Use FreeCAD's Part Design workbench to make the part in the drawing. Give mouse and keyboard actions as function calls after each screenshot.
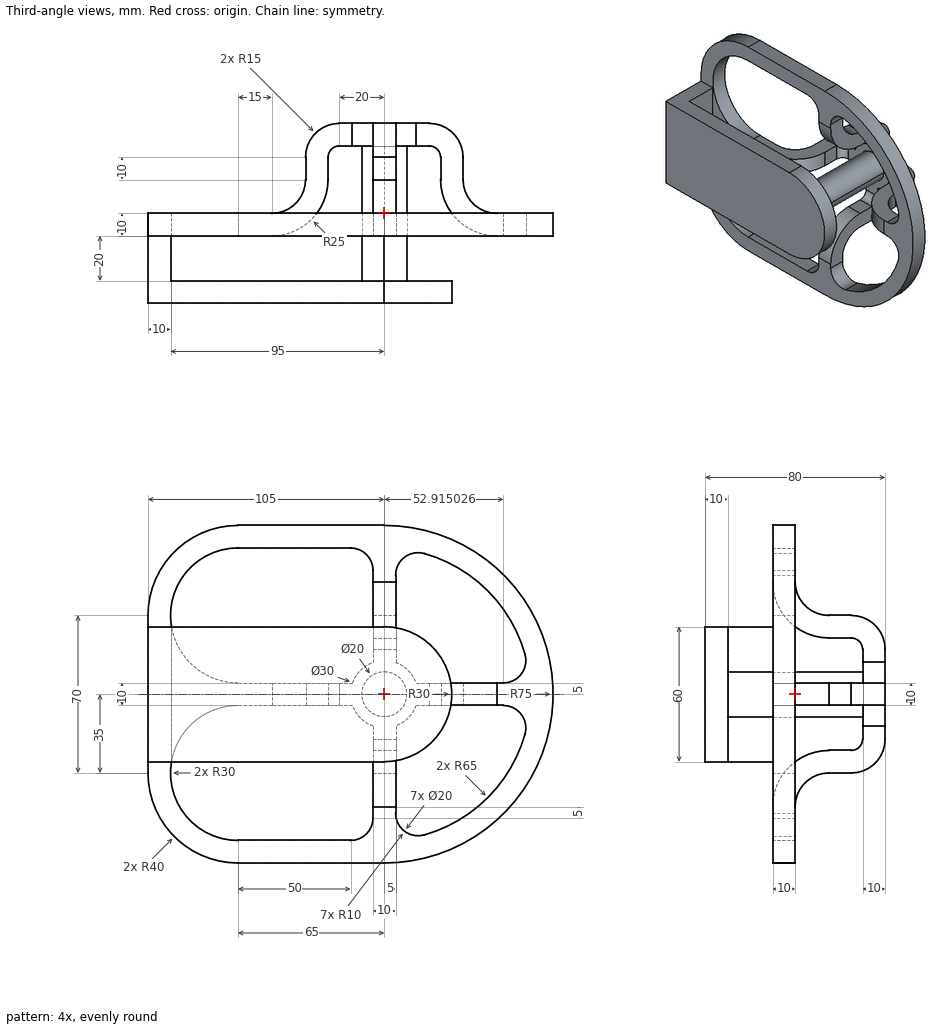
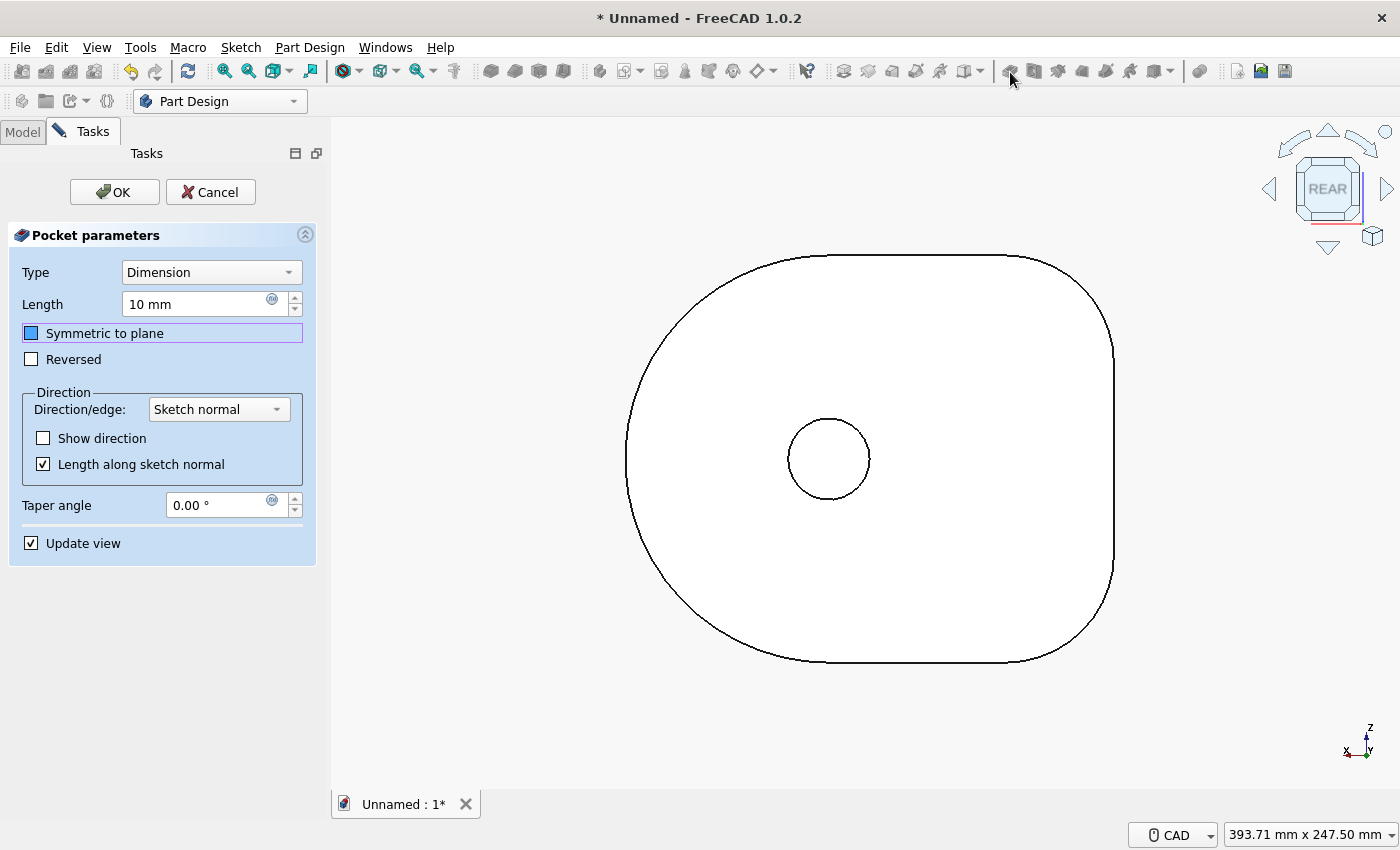
click(30, 359)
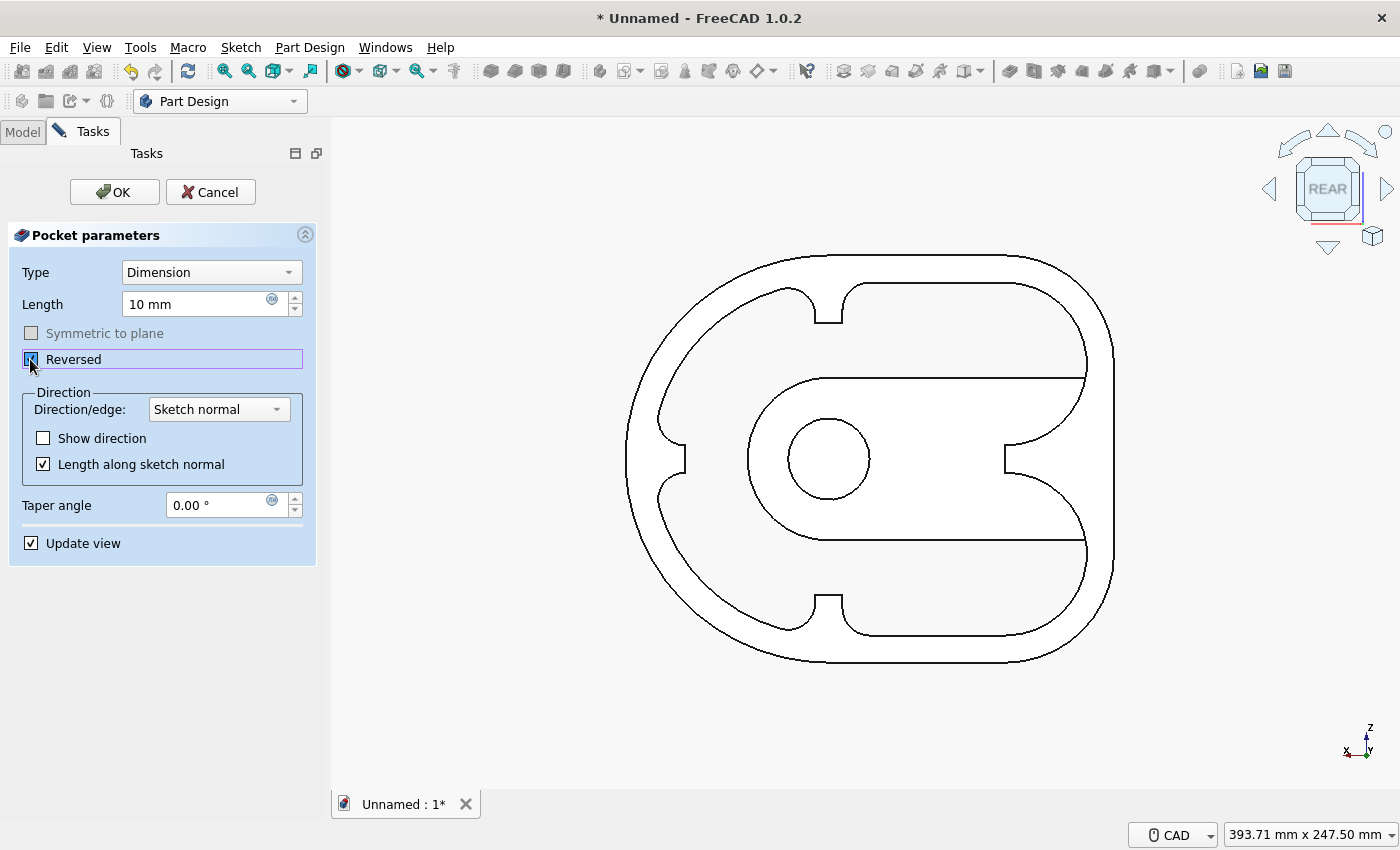
click(115, 192)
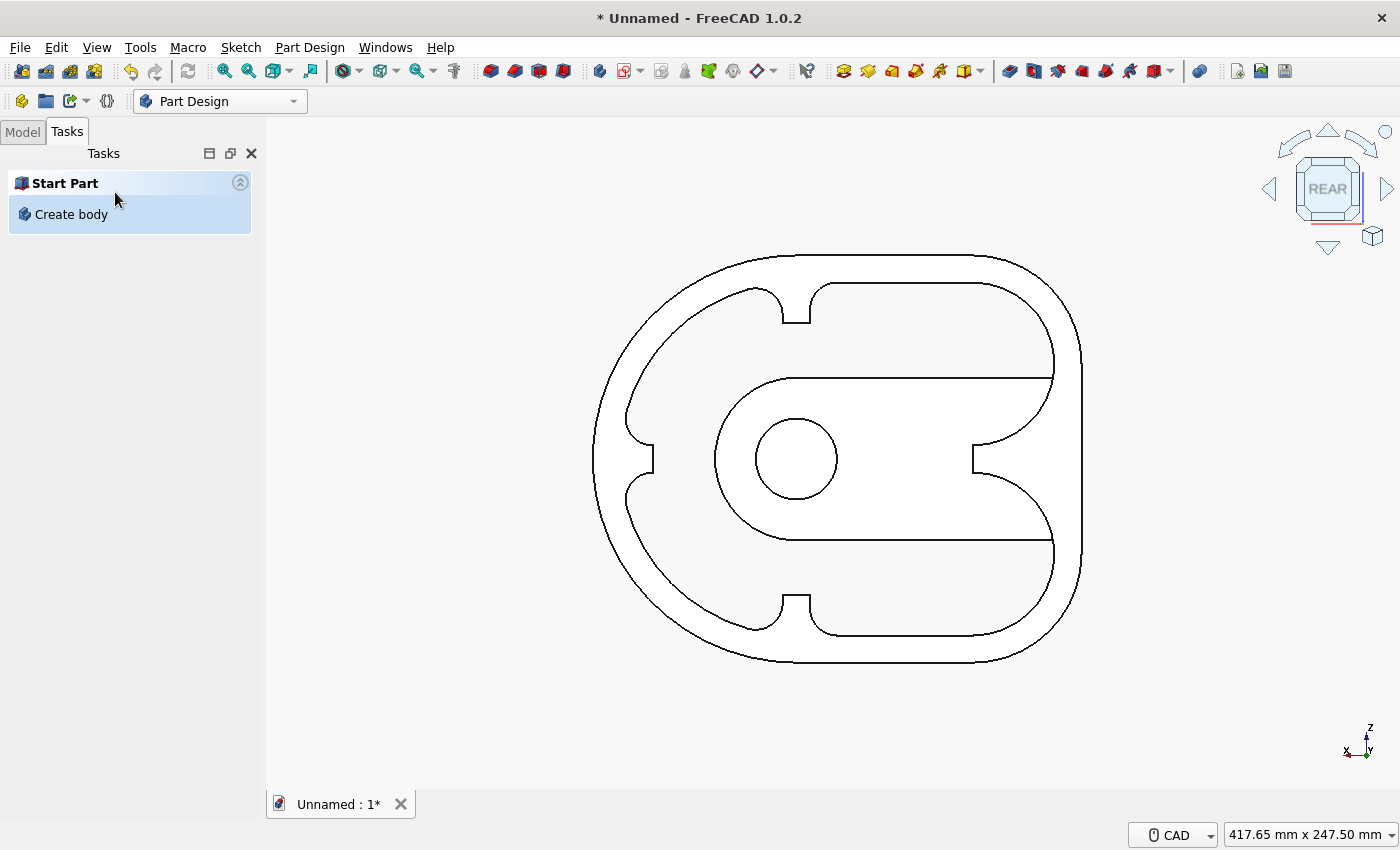
click(624, 72)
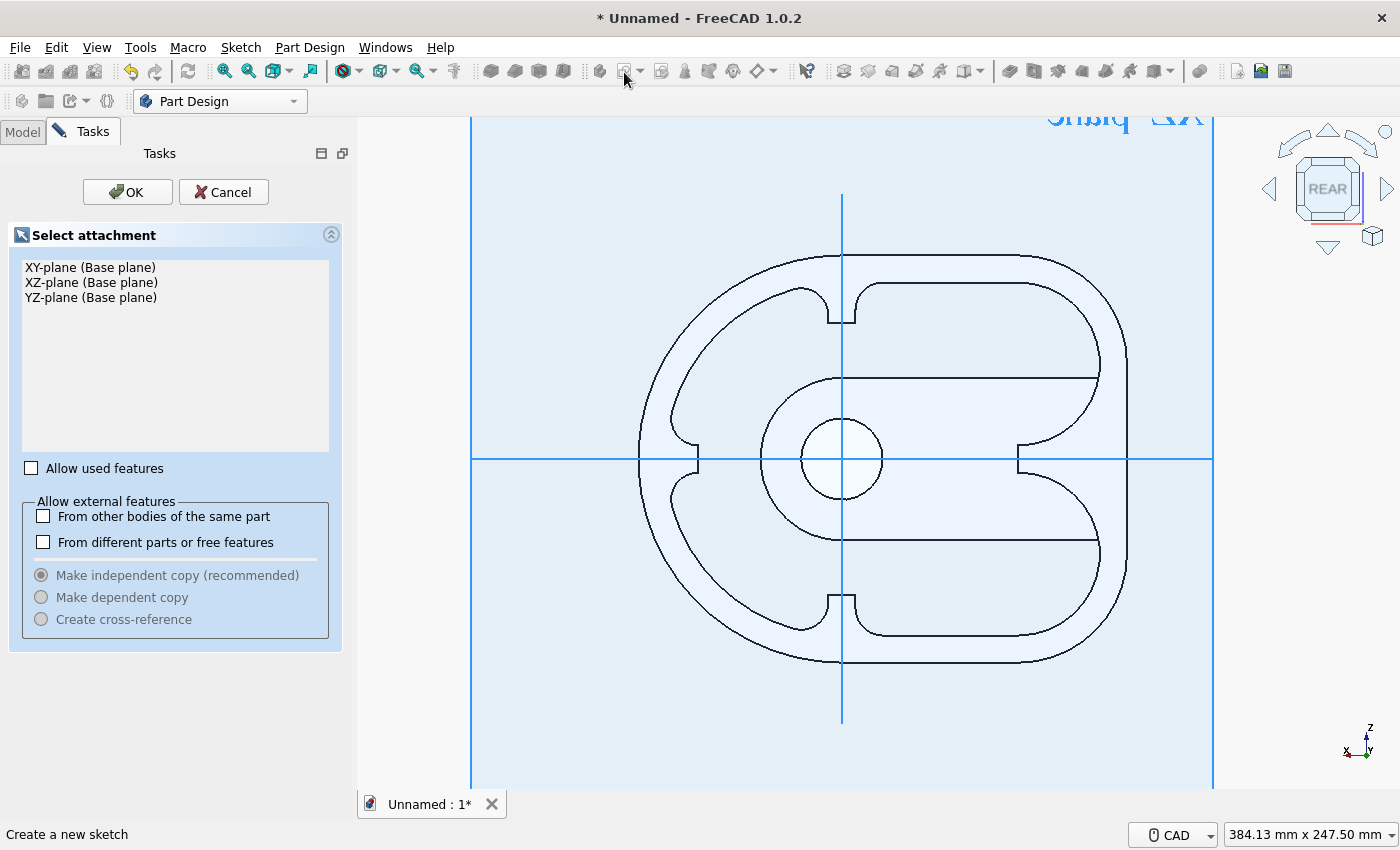
click(82, 268)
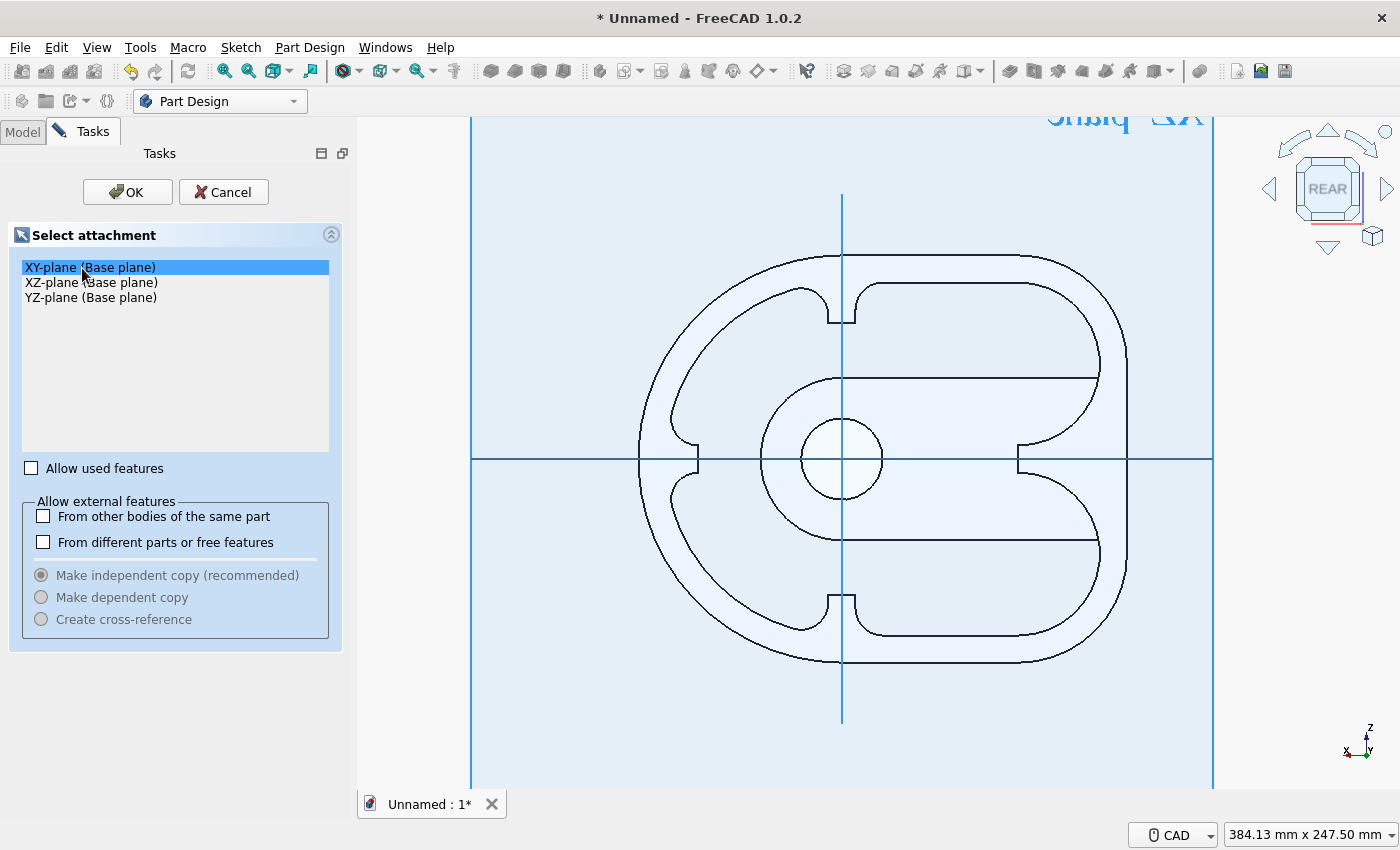
click(128, 192)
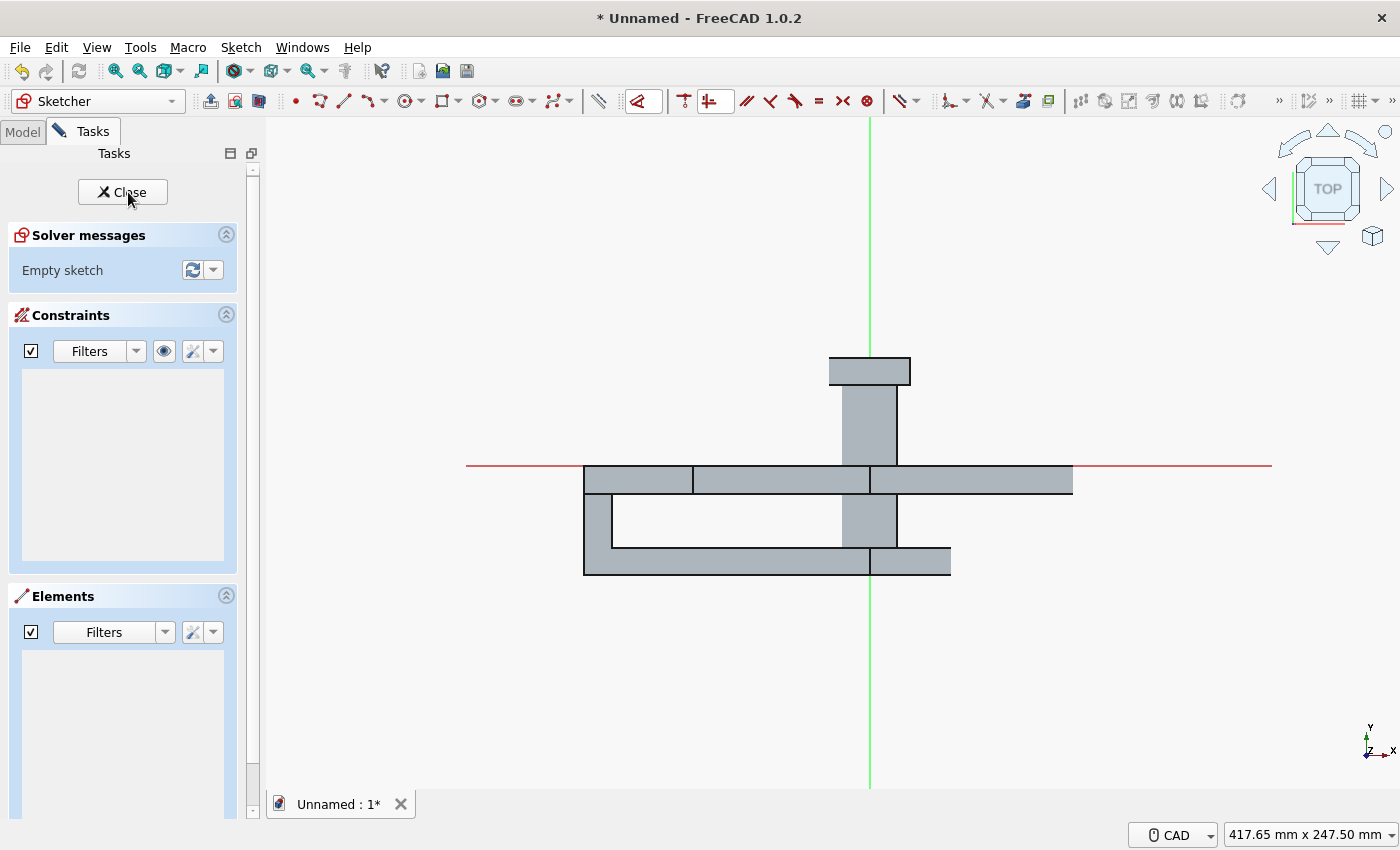
click(260, 102)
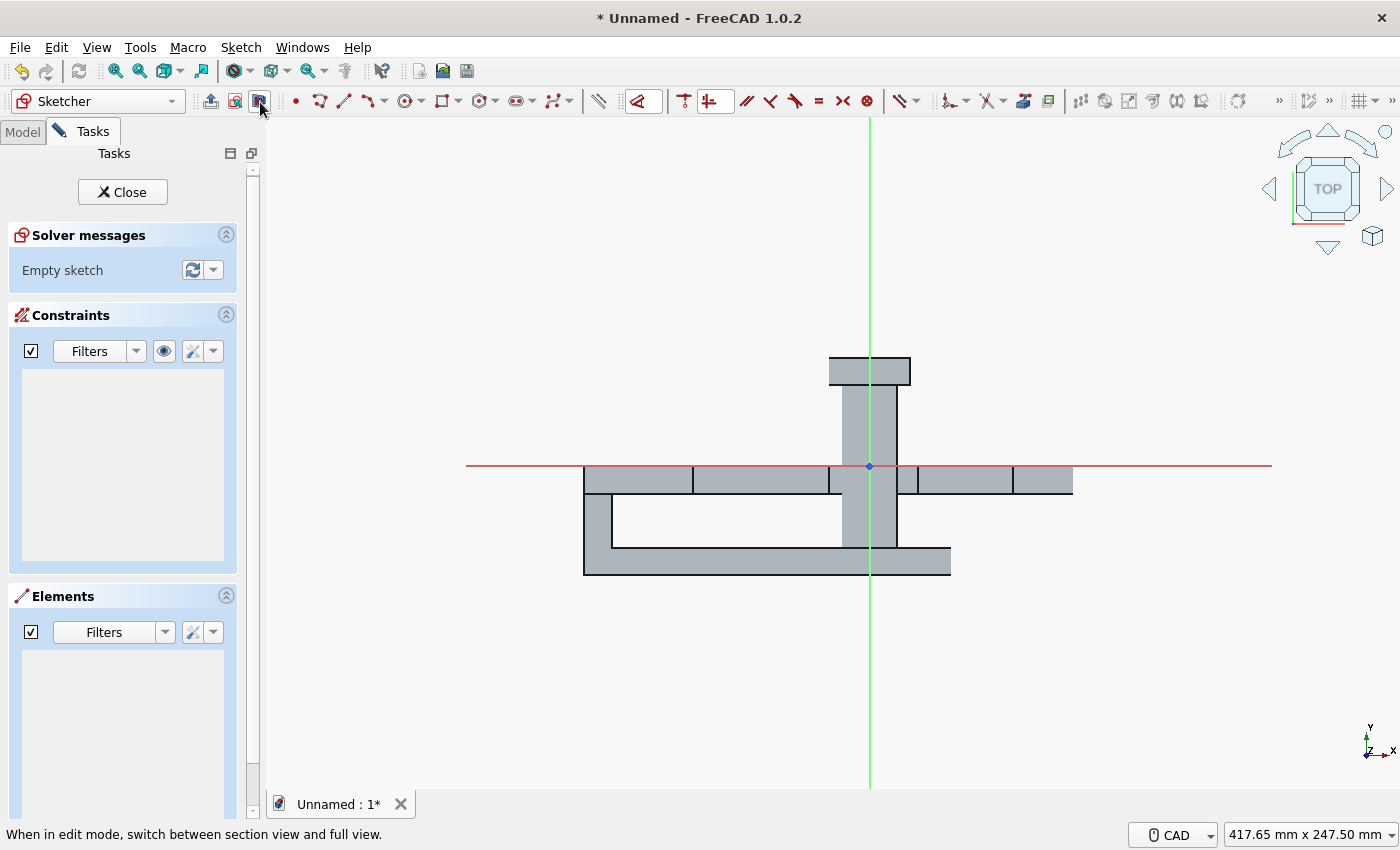
scroll(789, 414, up, 6)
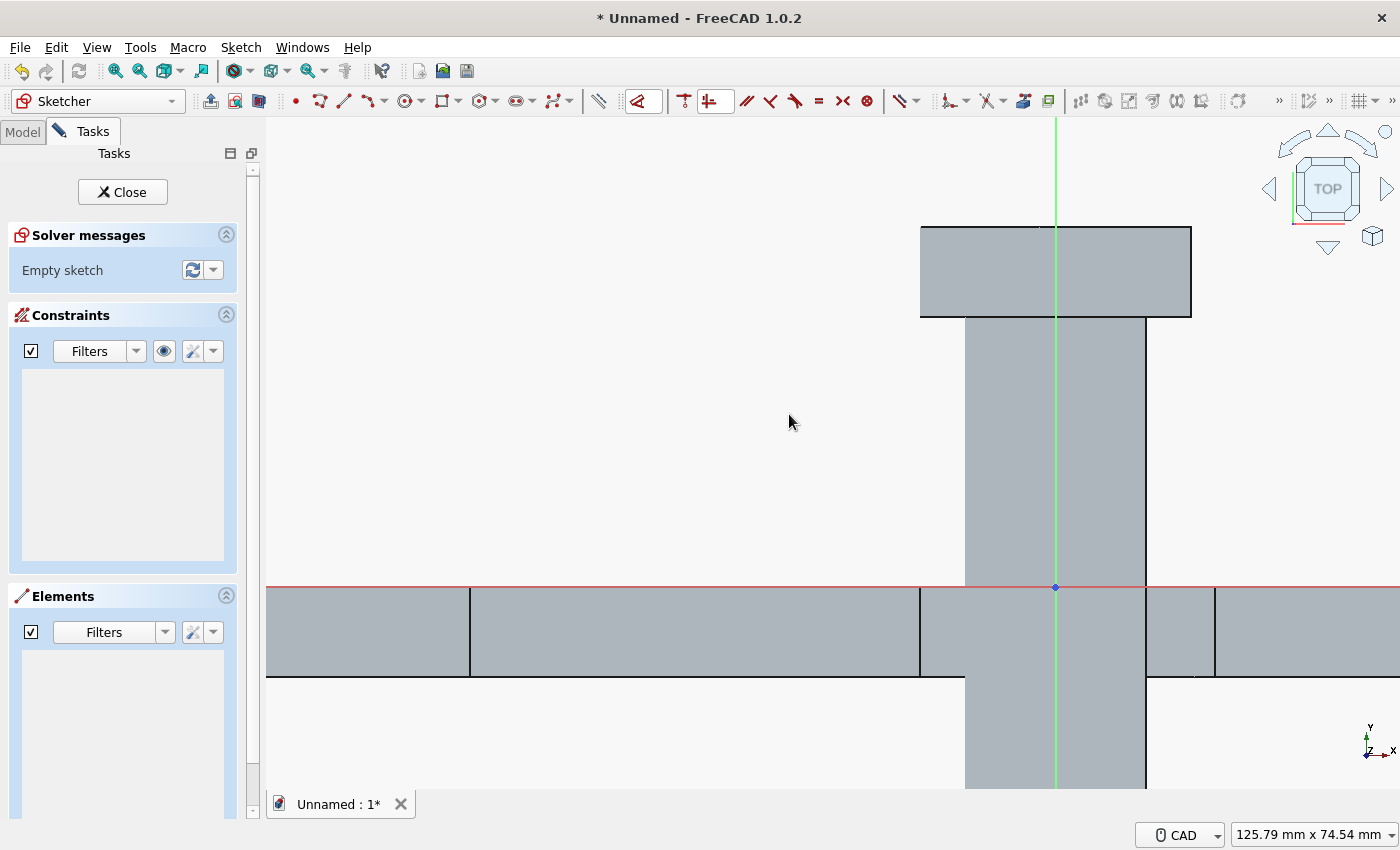
click(344, 102)